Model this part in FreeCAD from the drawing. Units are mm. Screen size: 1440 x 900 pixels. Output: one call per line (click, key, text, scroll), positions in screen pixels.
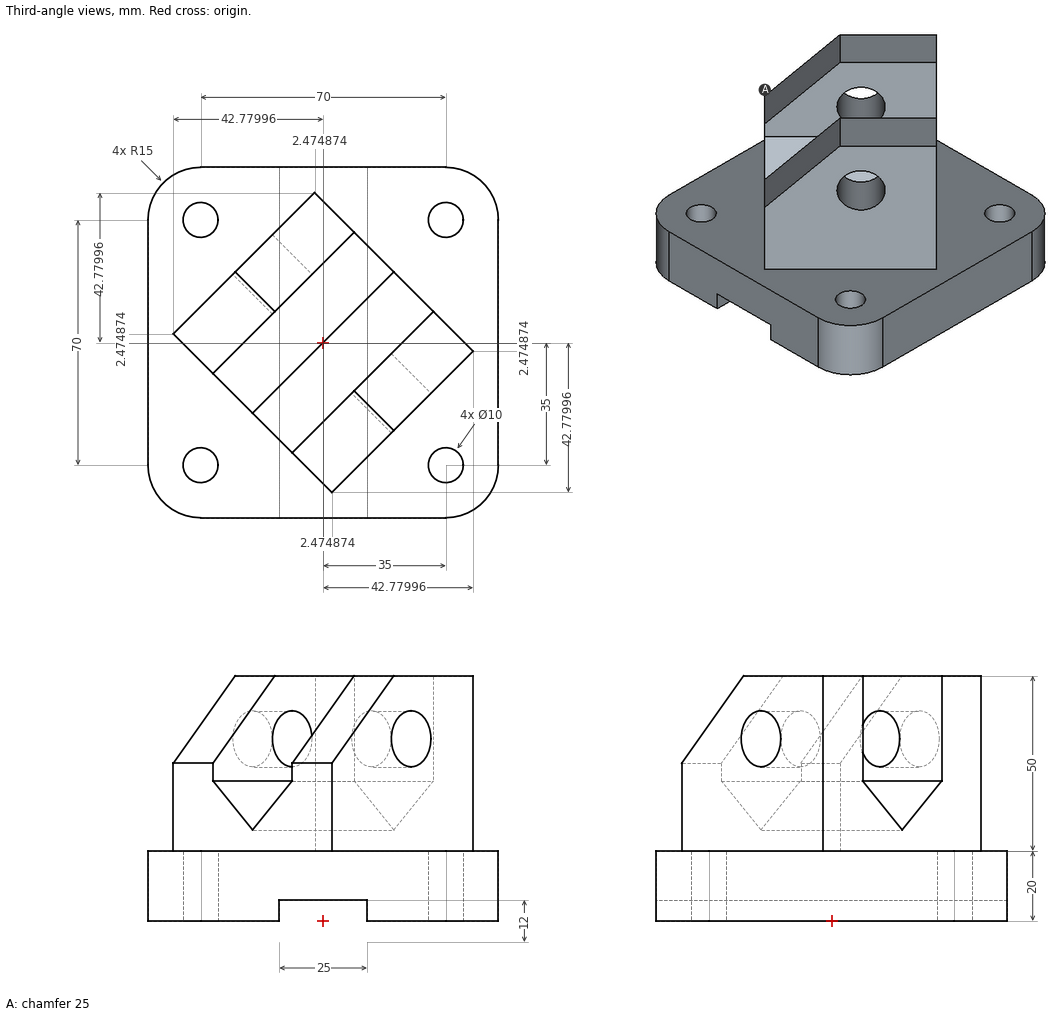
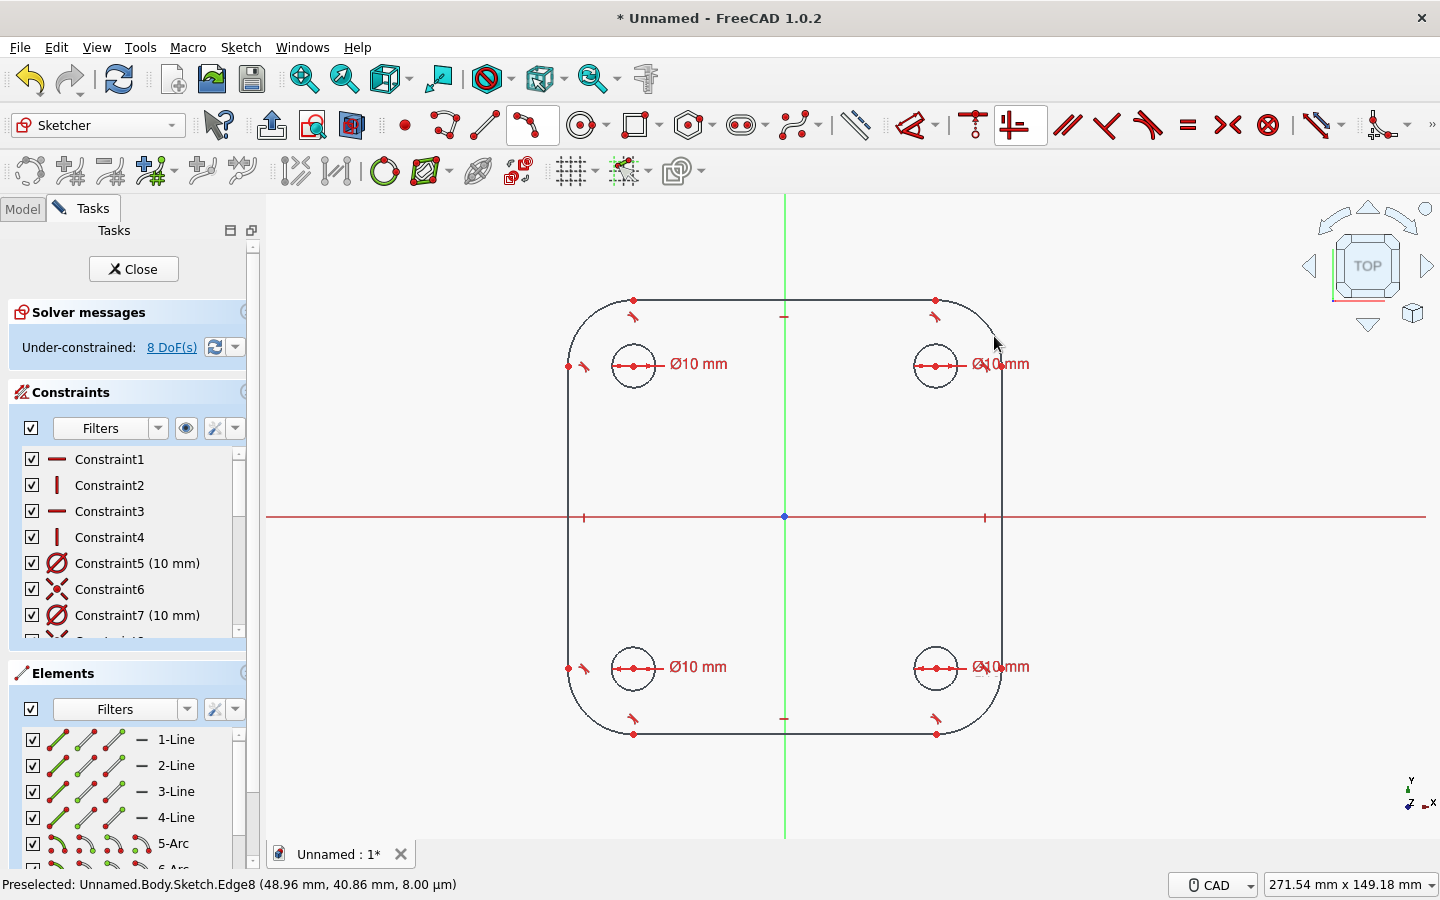
click(604, 307)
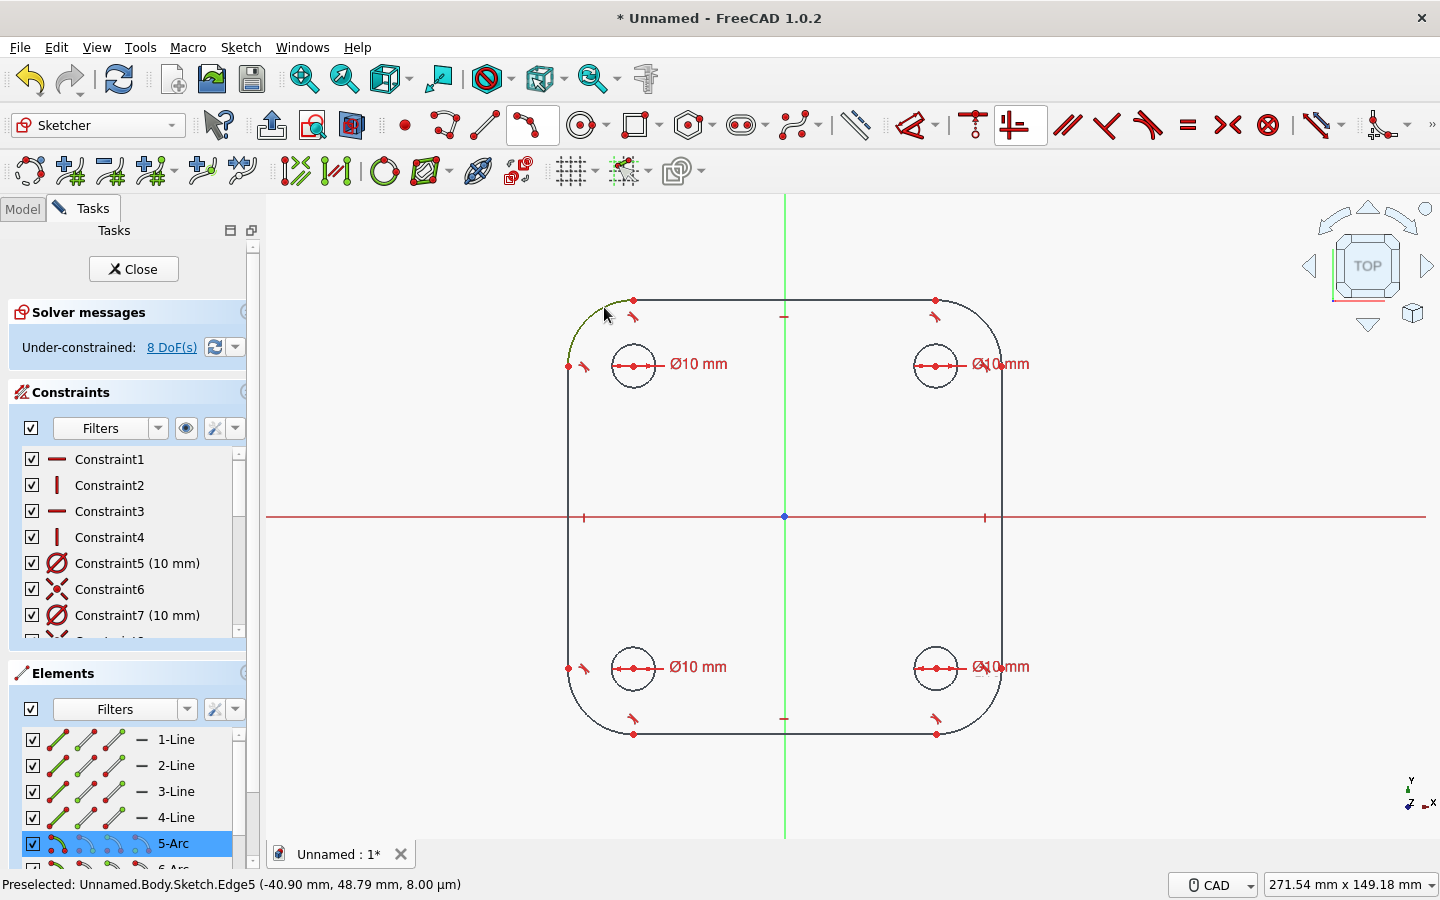
click(575, 699)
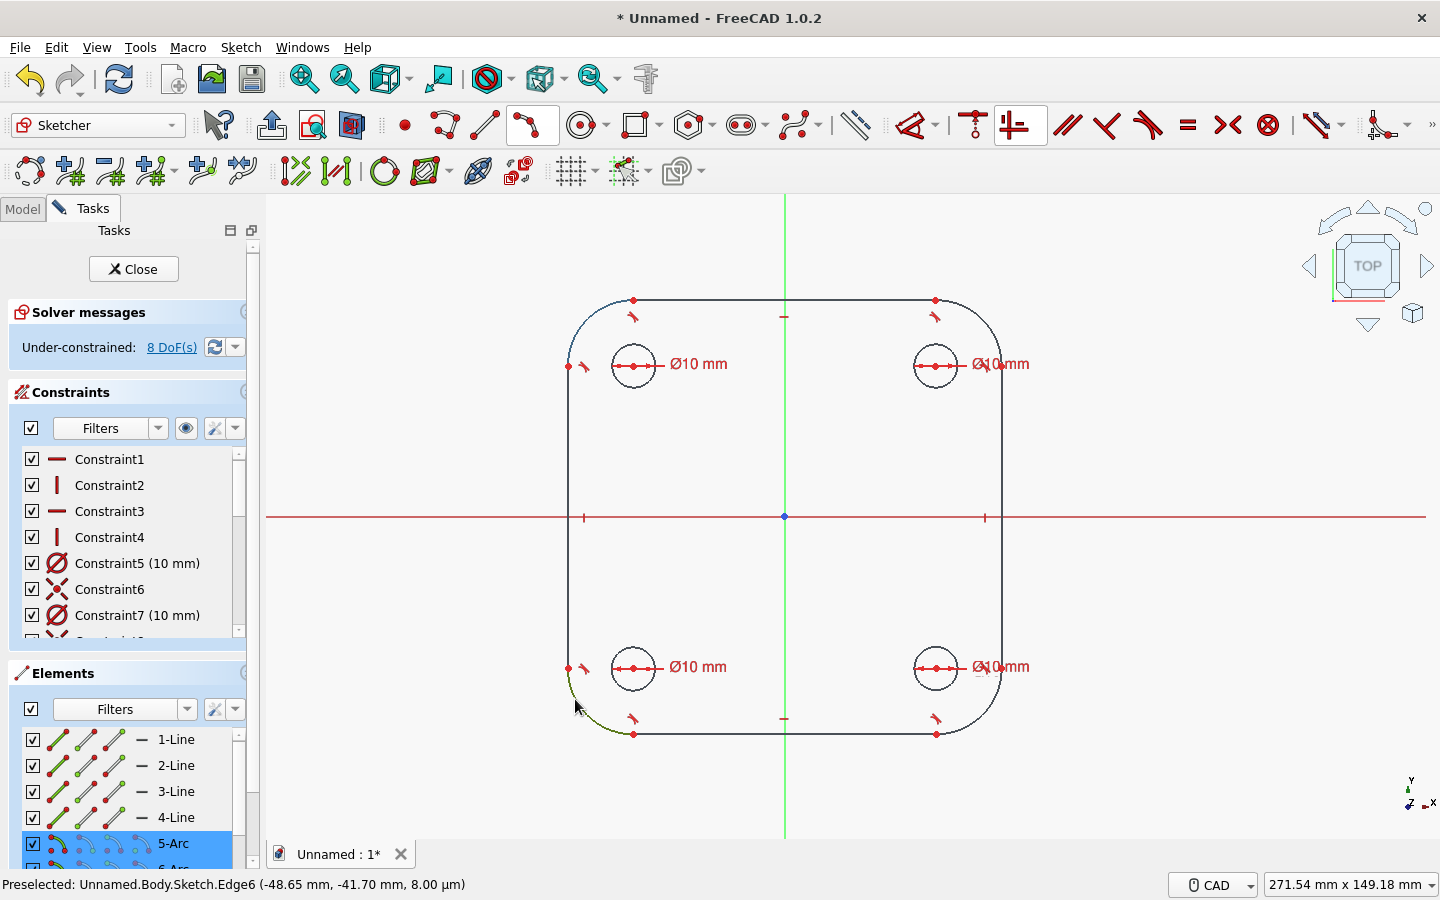
click(966, 727)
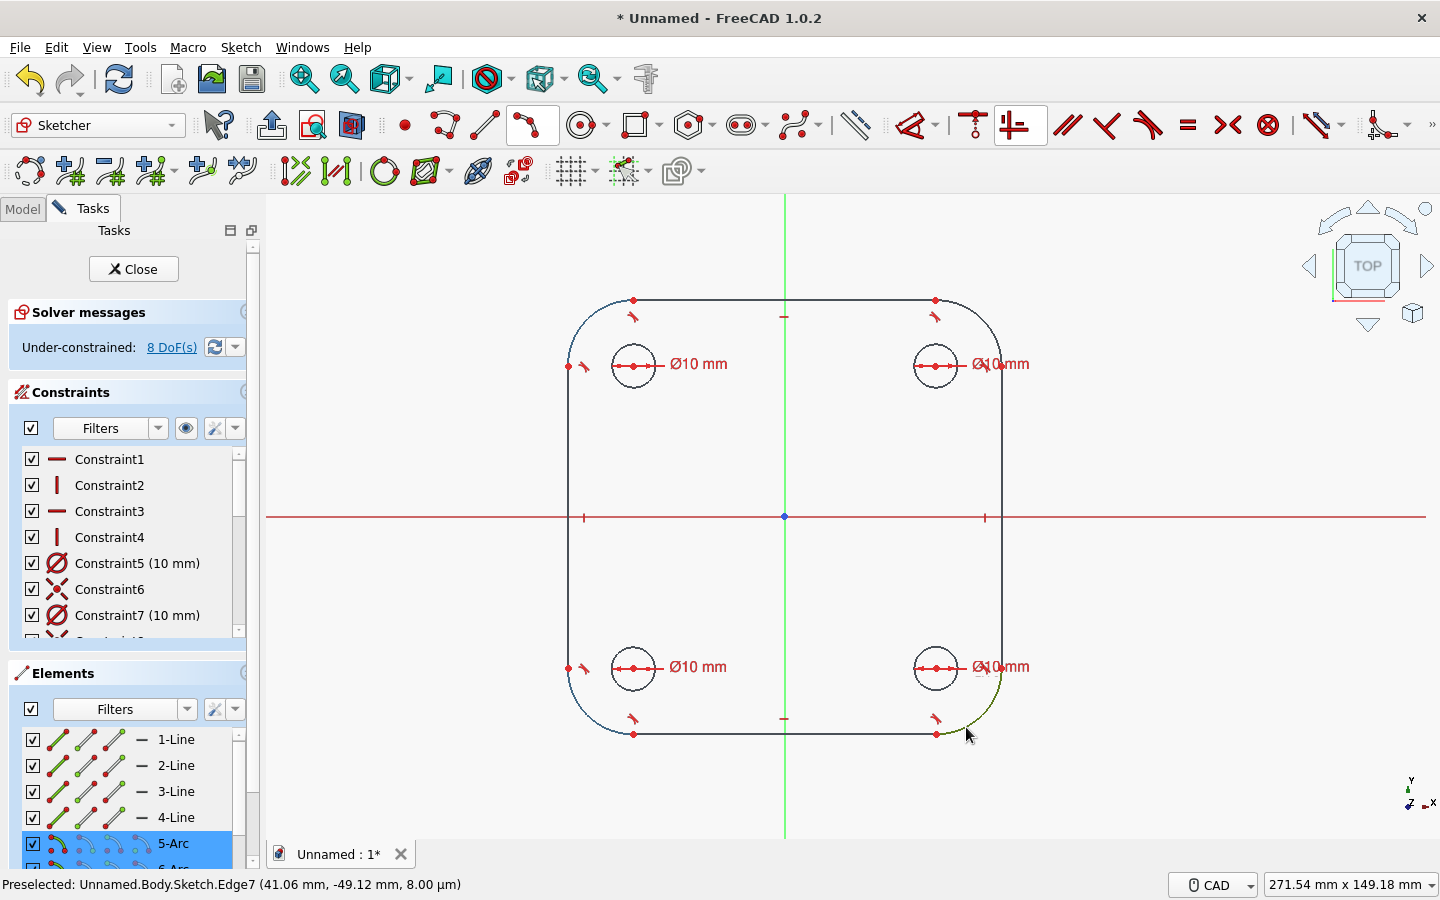
click(994, 336)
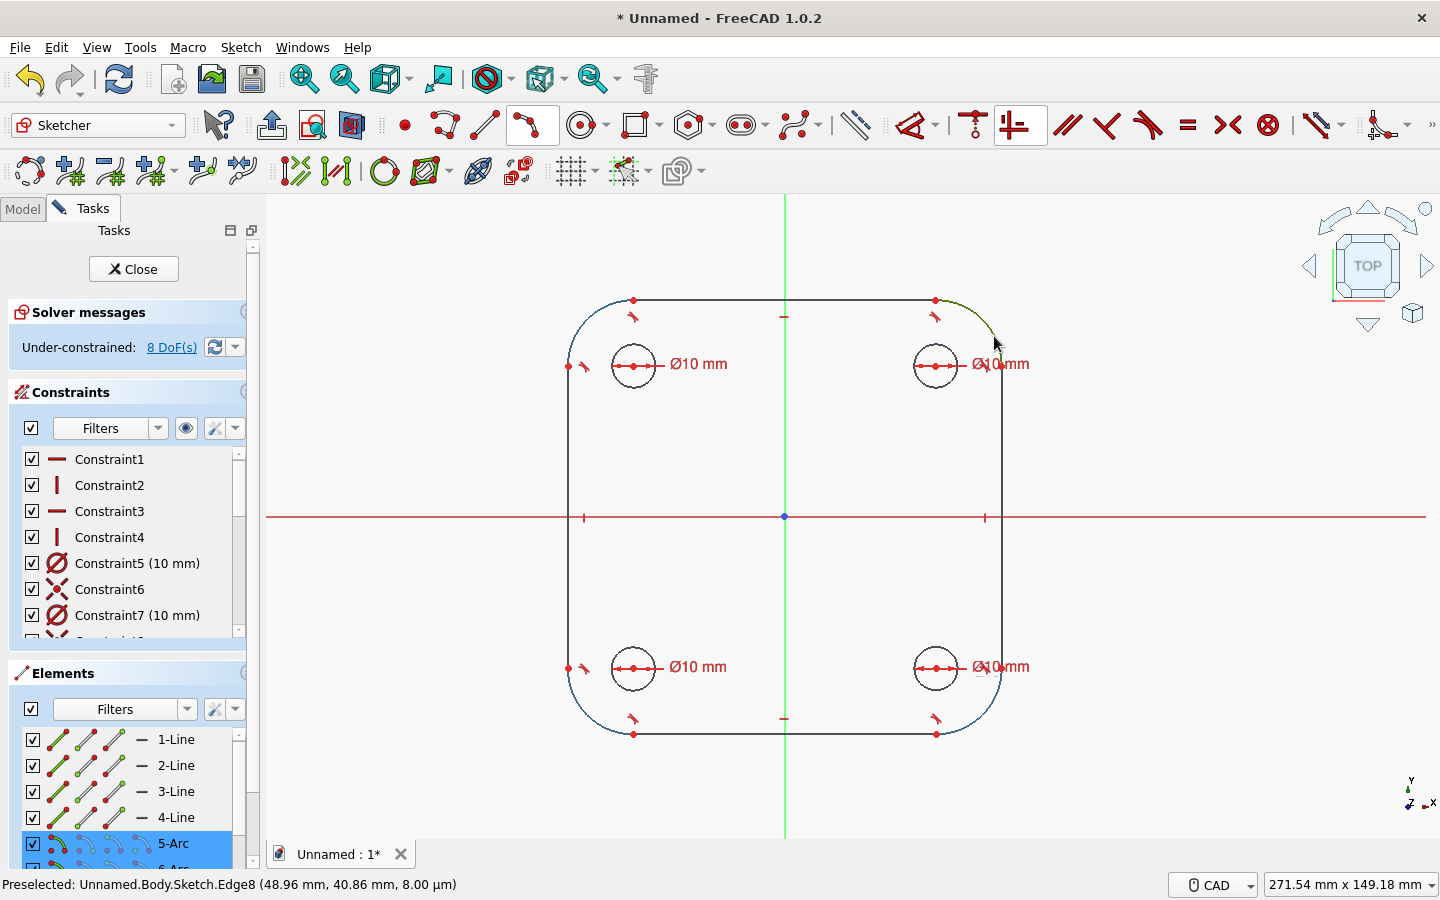
key(e)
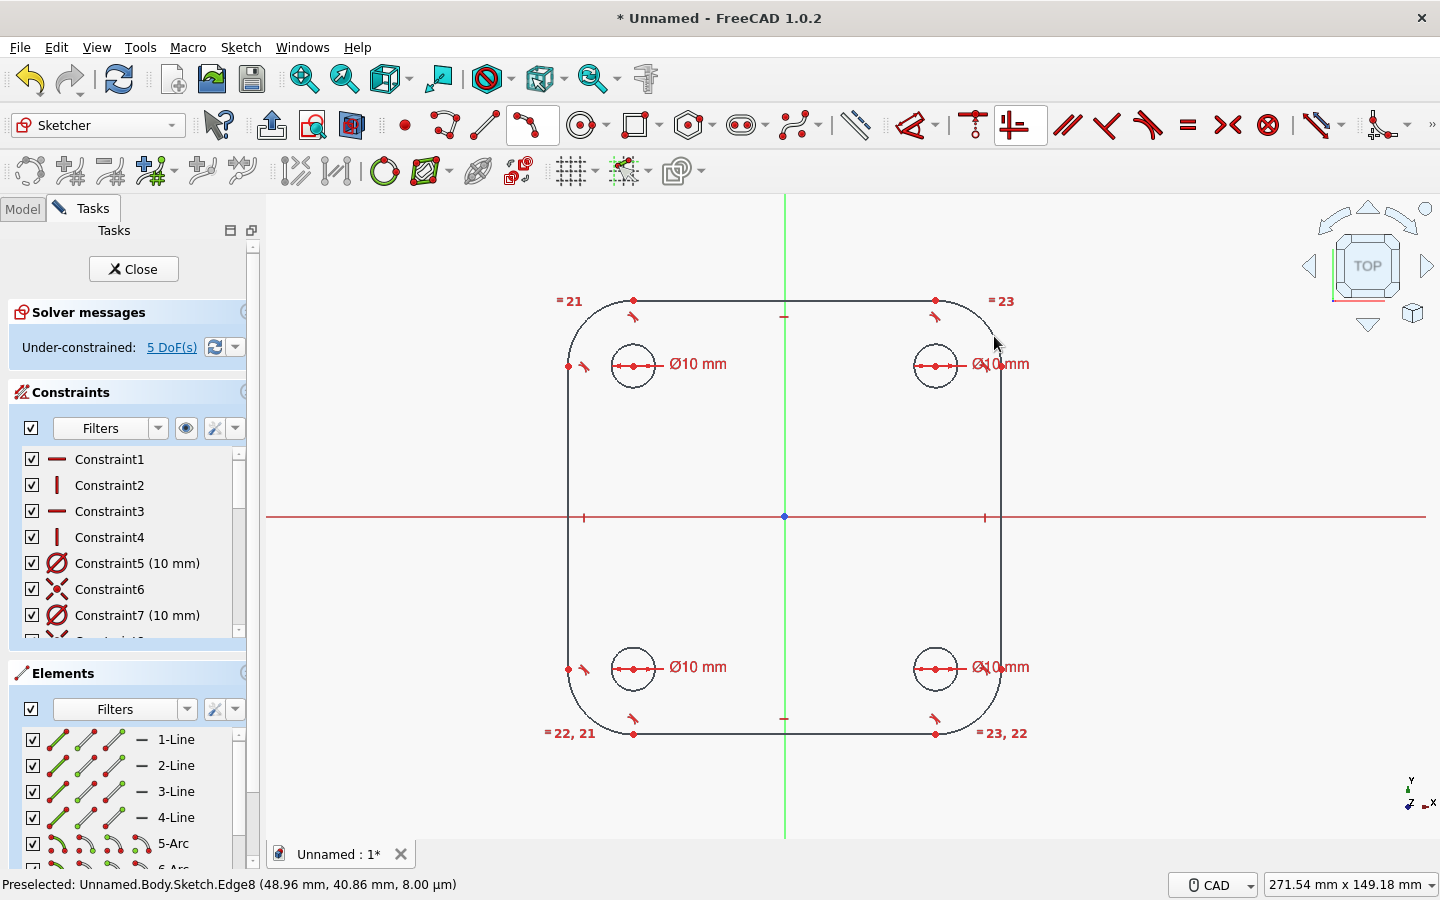
key(d)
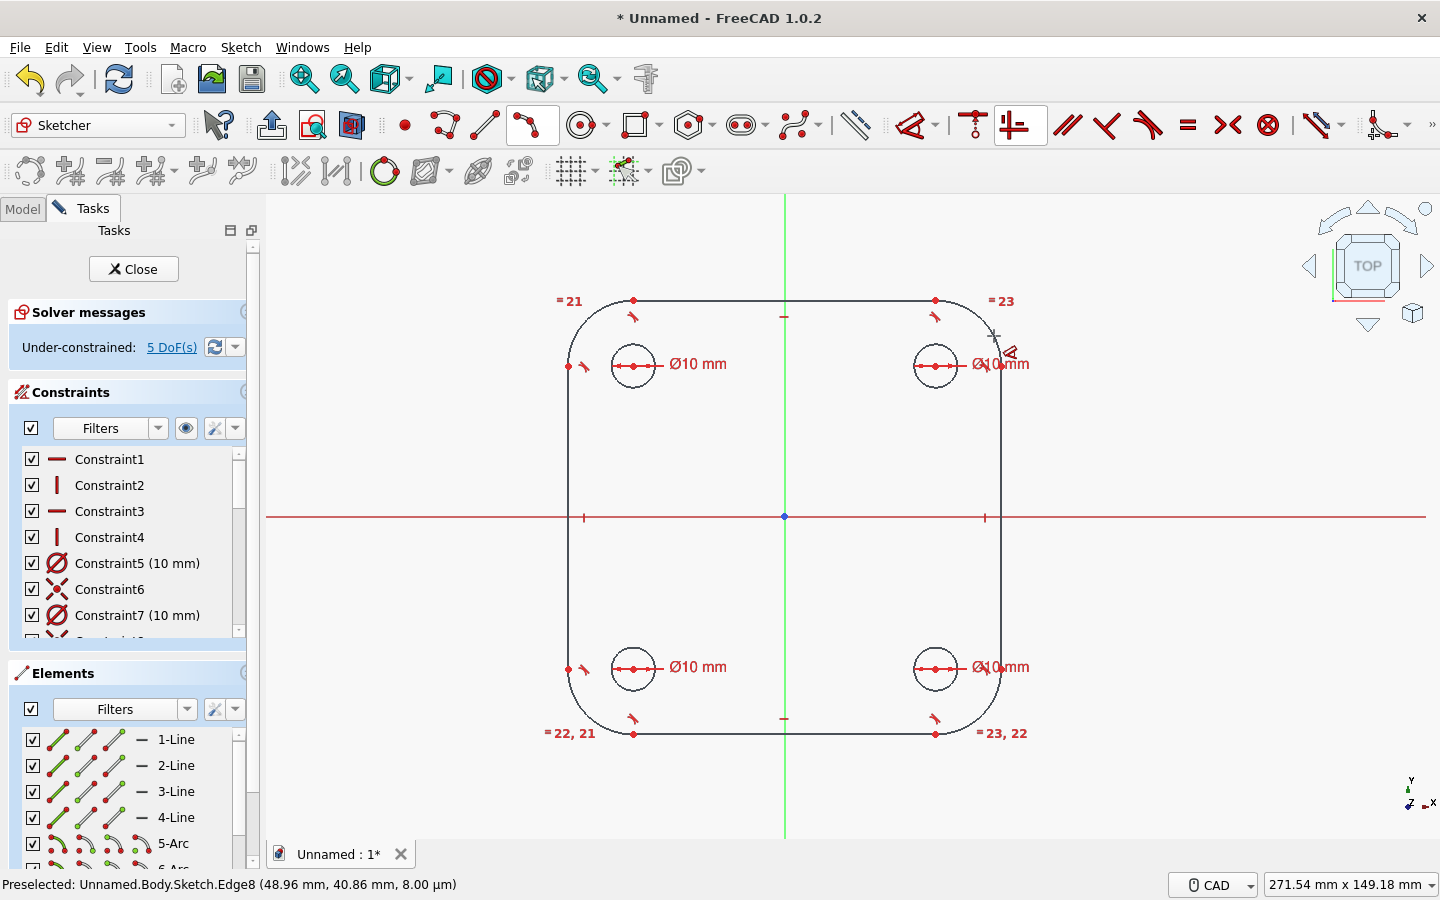
click(604, 308)
click(590, 279)